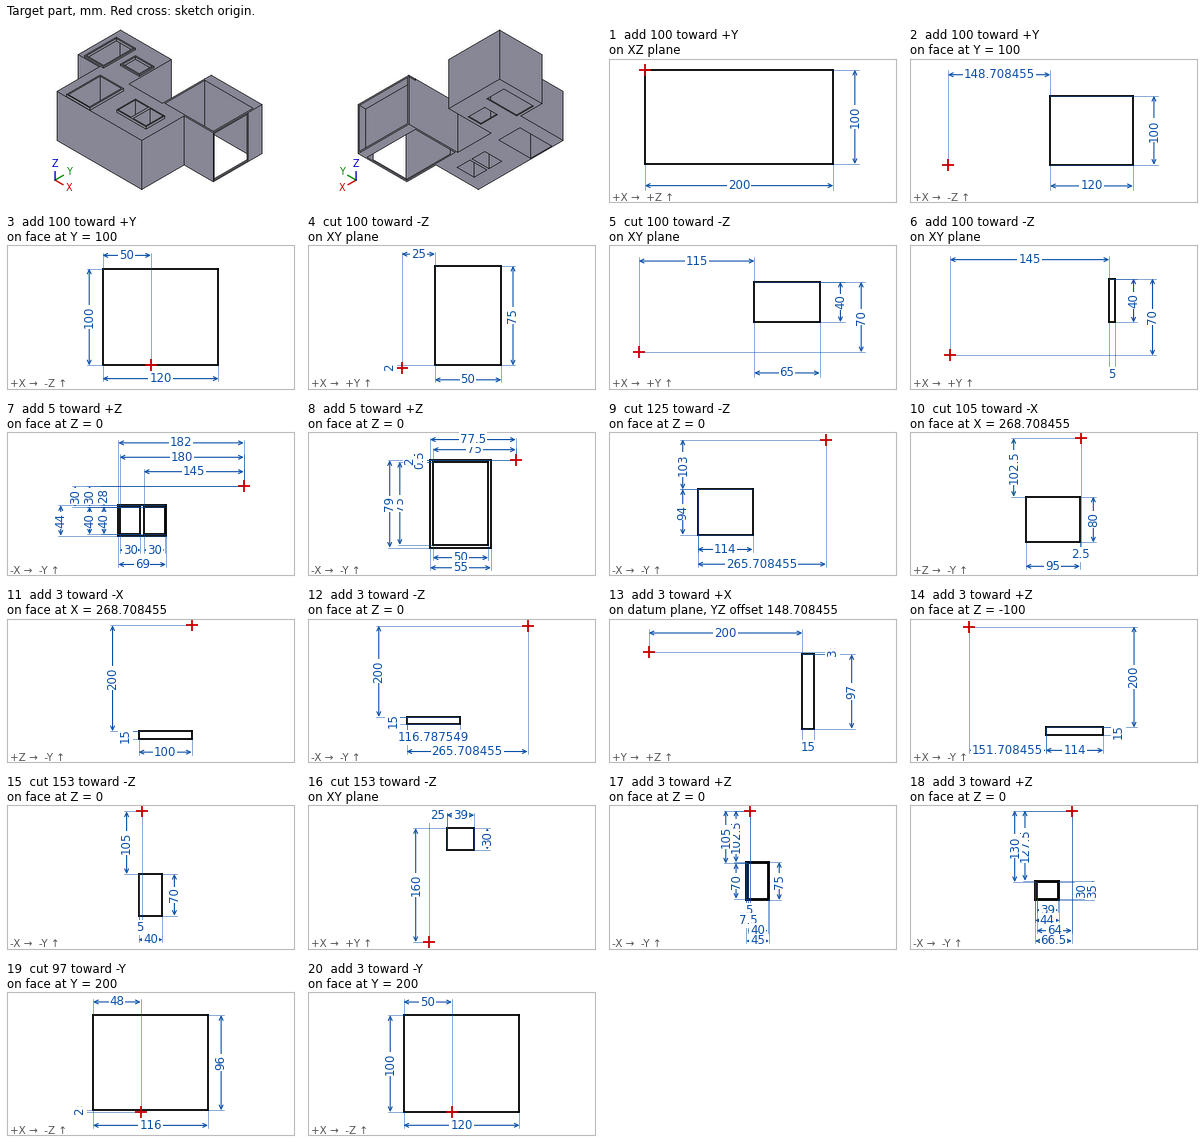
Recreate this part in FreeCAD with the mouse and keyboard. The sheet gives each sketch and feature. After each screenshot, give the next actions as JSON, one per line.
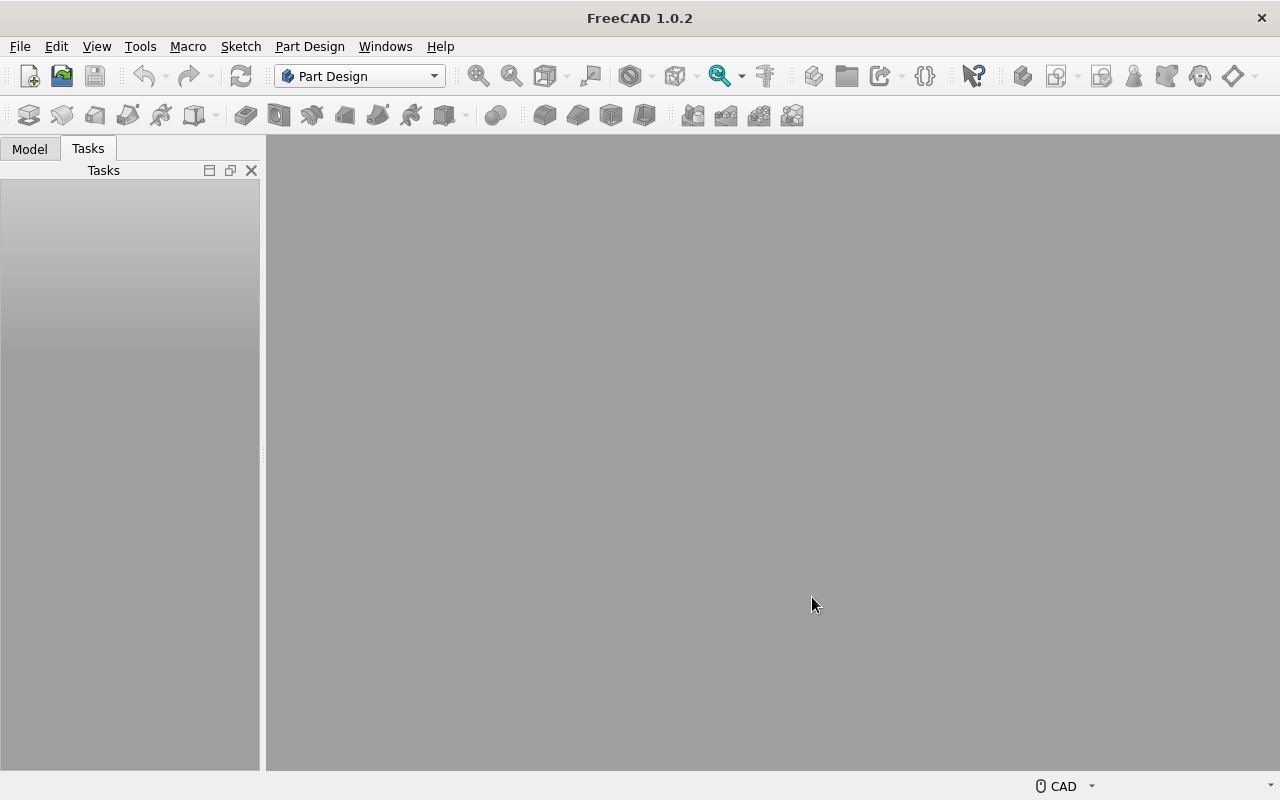
{"action": "left_click", "coordinate": [29, 76]}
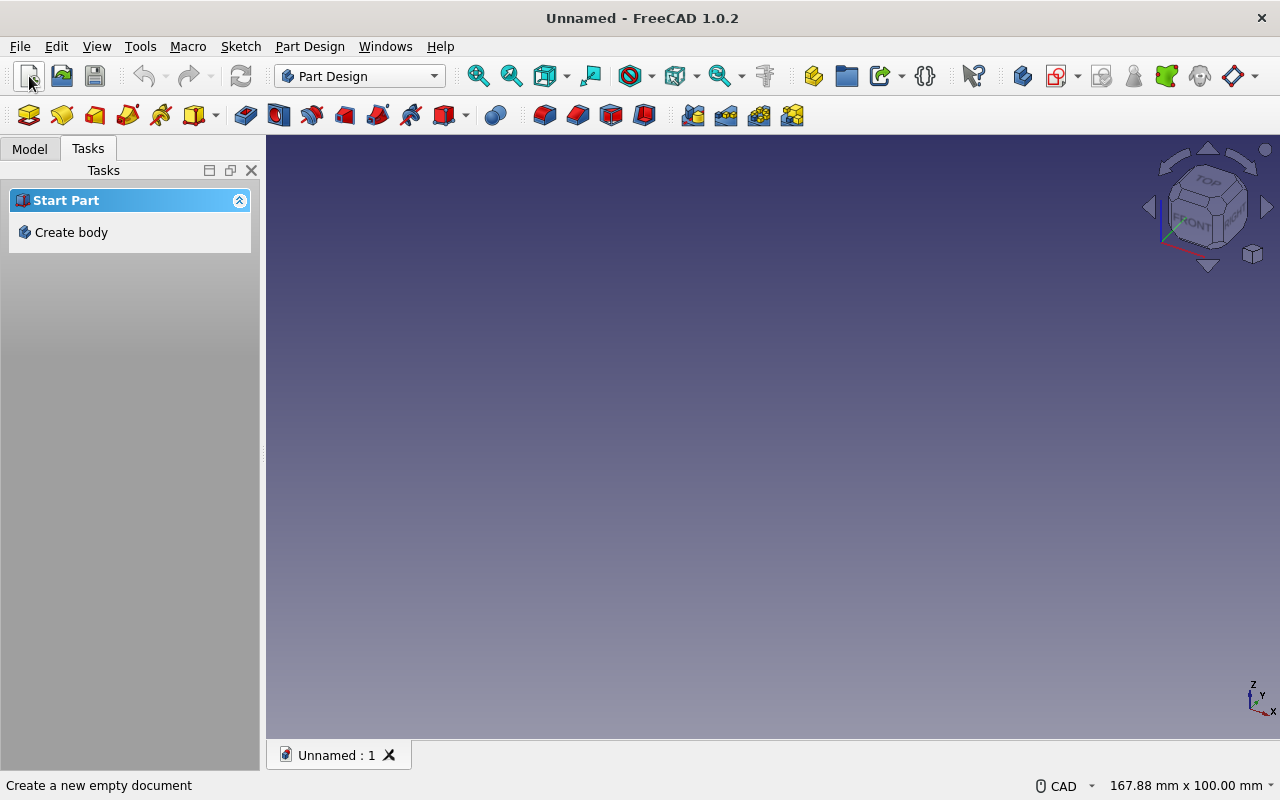
{"action": "left_click", "coordinate": [1056, 76]}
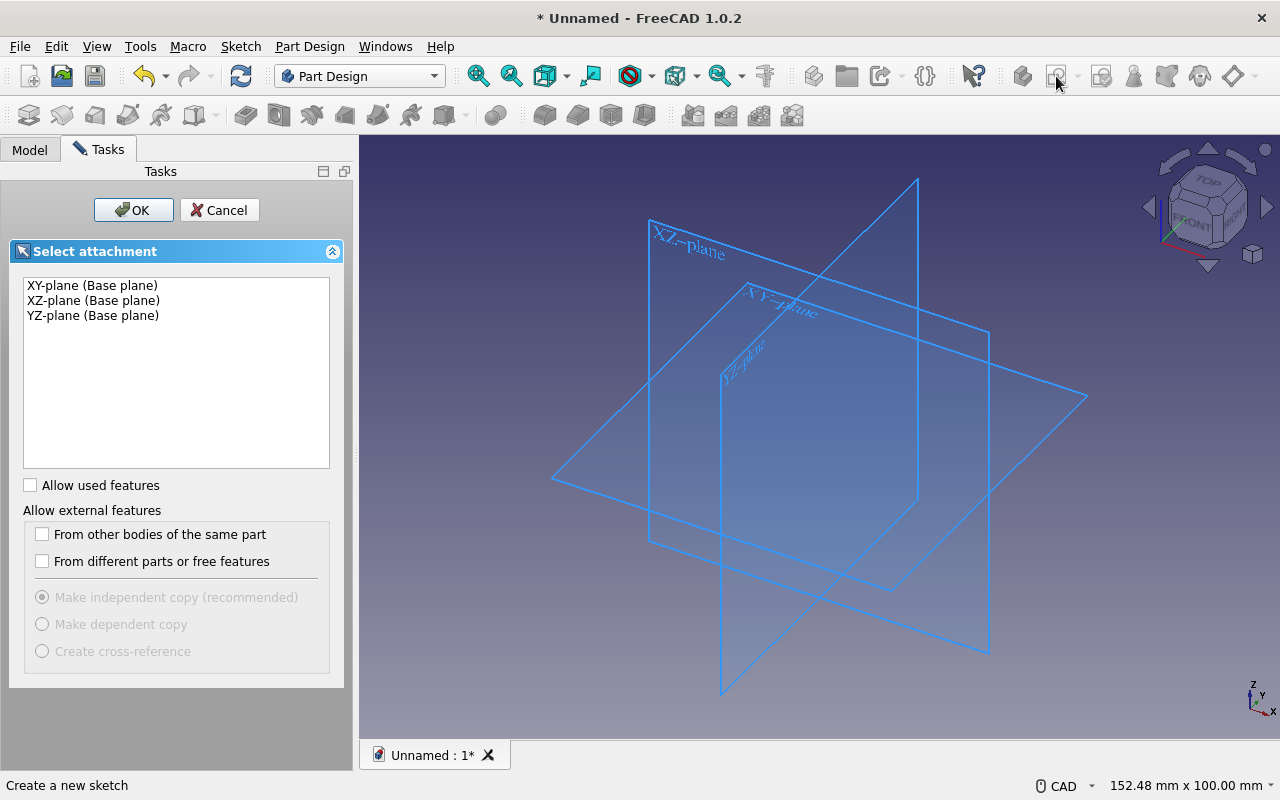
{"action": "left_click", "coordinate": [84, 300]}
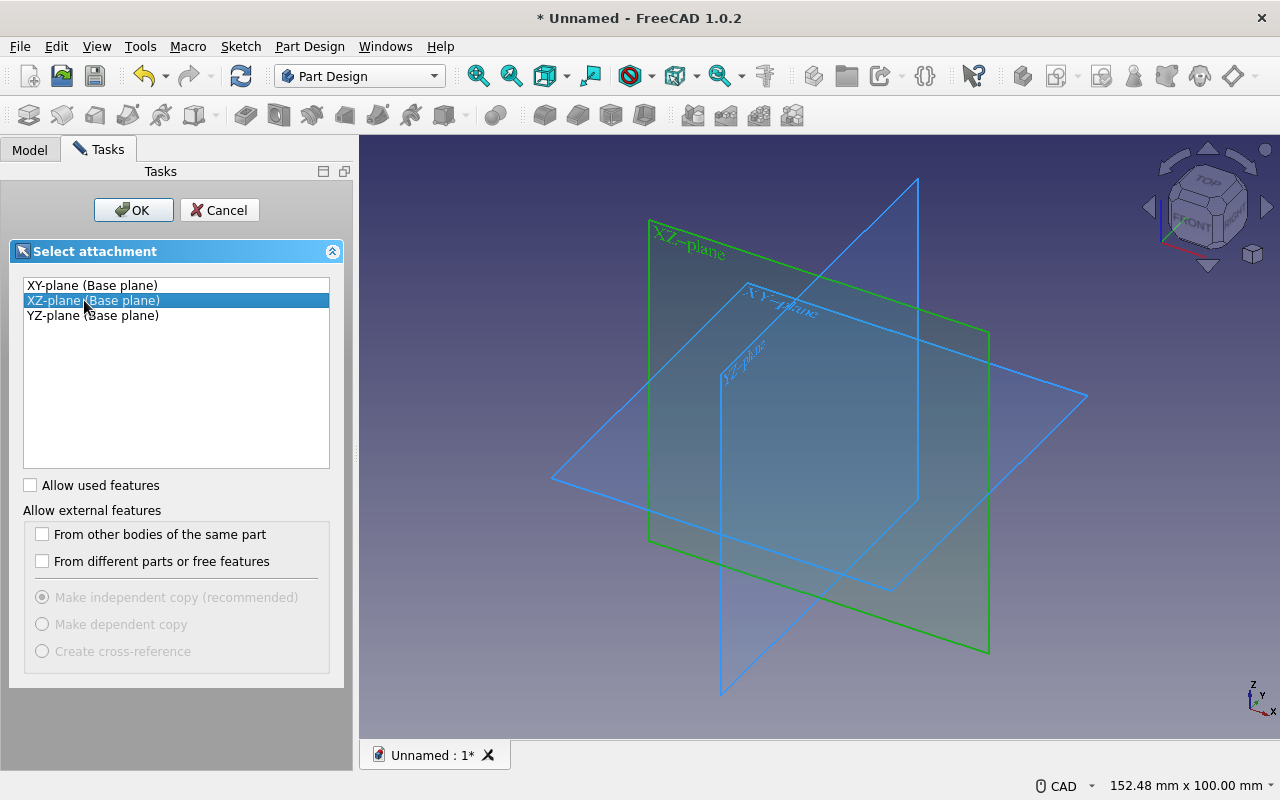
{"action": "left_click", "coordinate": [134, 210]}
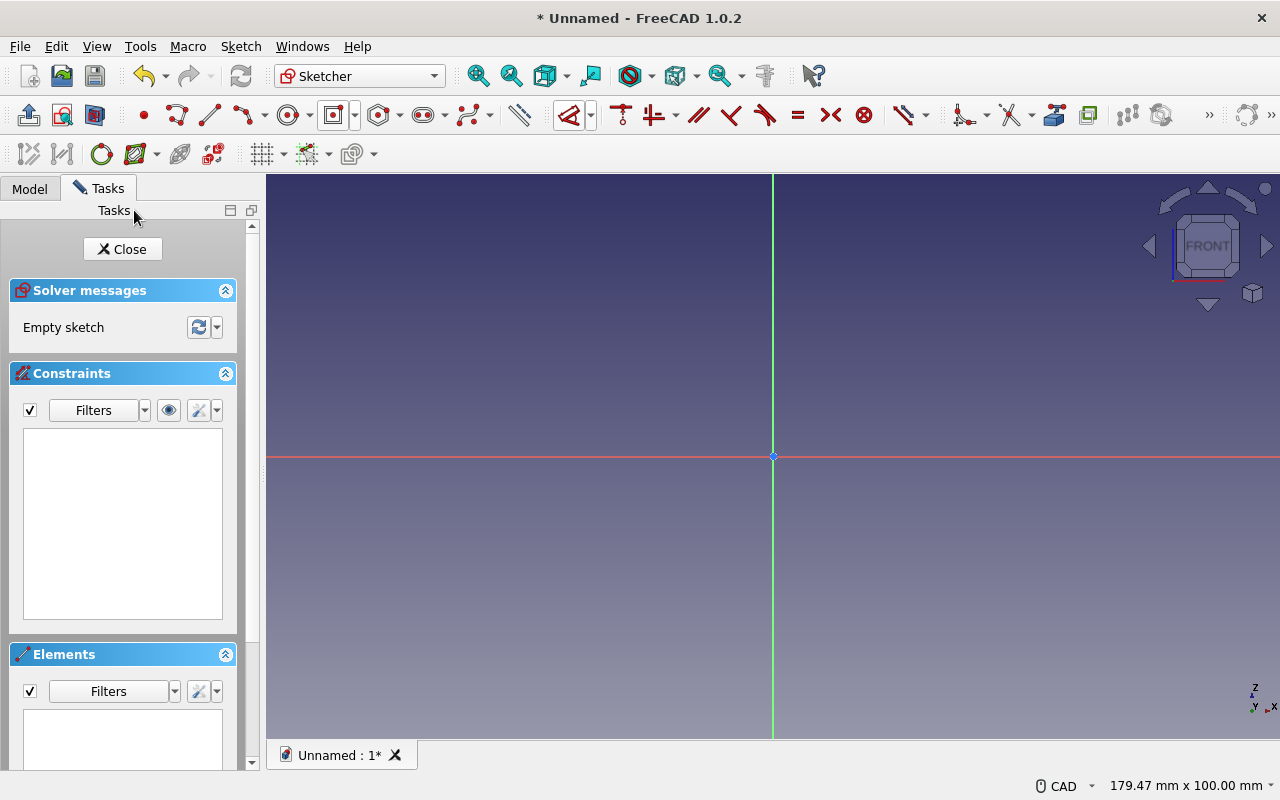
{"action": "scroll", "coordinate": [294, 226], "scroll_direction": "down", "scroll_amount": 4}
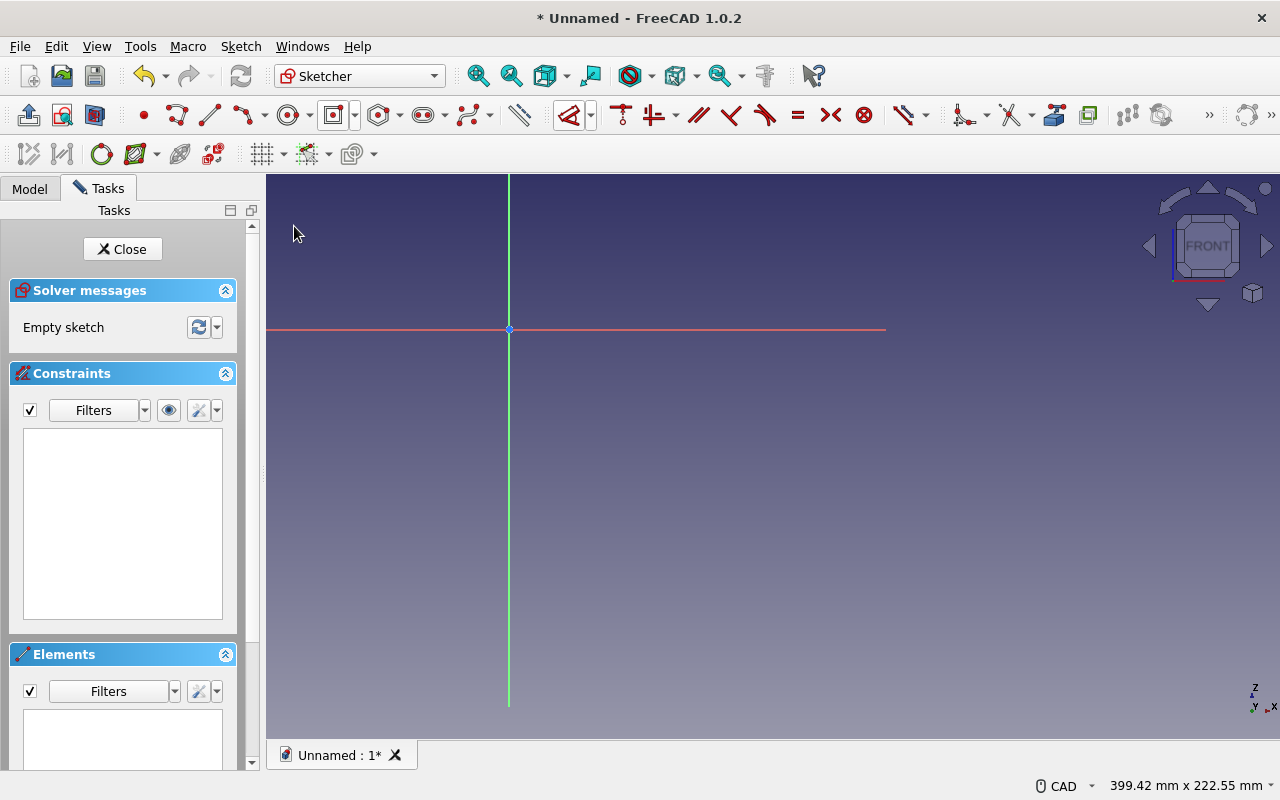
{"action": "key", "text": "g r"}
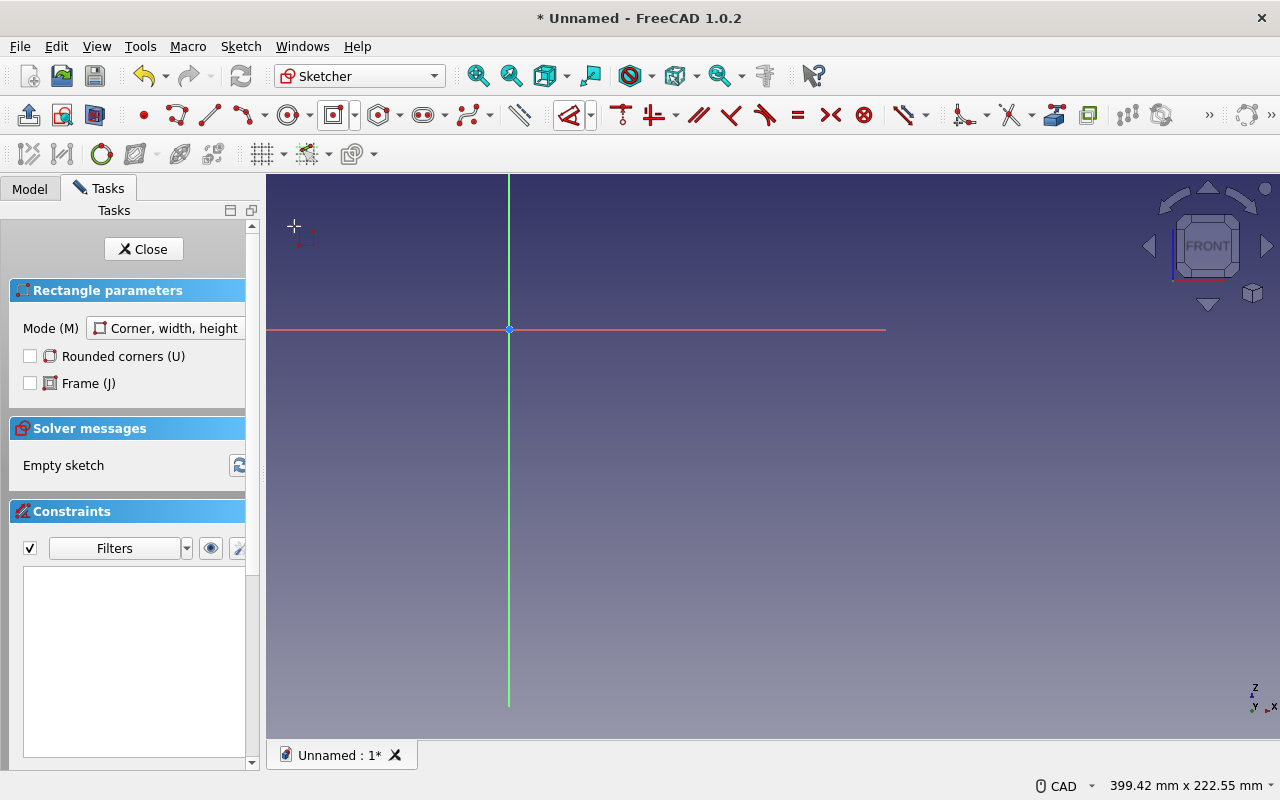
{"action": "left_click", "coordinate": [509, 330]}
{"action": "mouse_move", "coordinate": [1017, 583]}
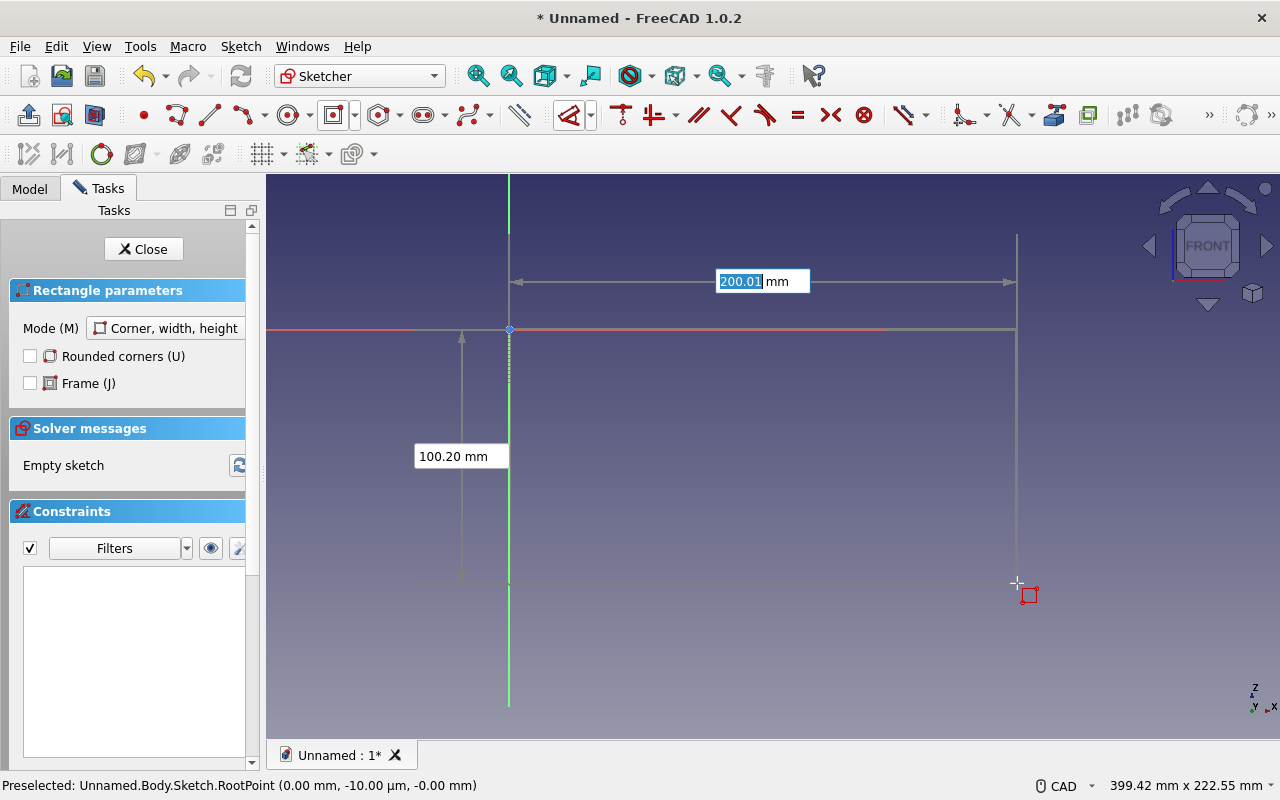
{"action": "type", "text": "200"}
{"action": "key", "text": "Tab"}
{"action": "type", "text": "100"}
{"action": "key", "text": "Return"}
{"action": "key", "text": "Escape"}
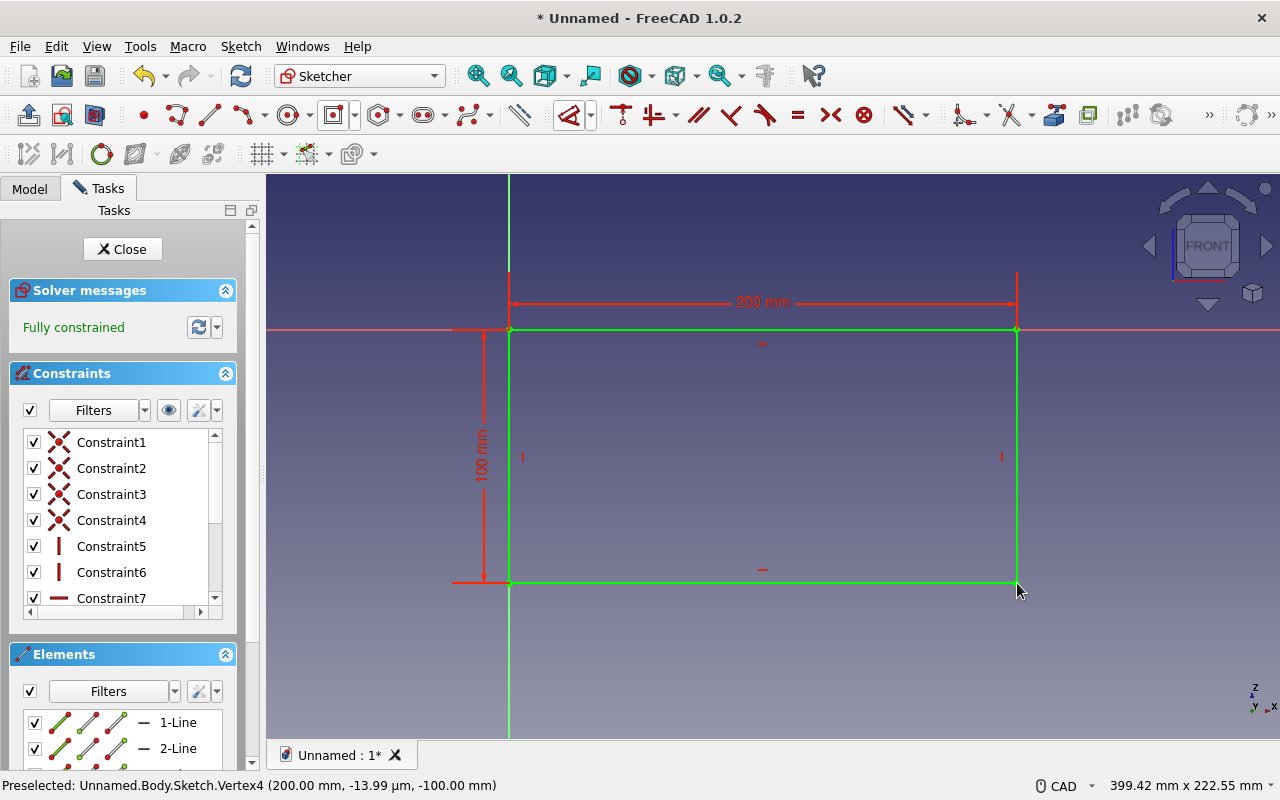
{"action": "left_click", "coordinate": [123, 249]}